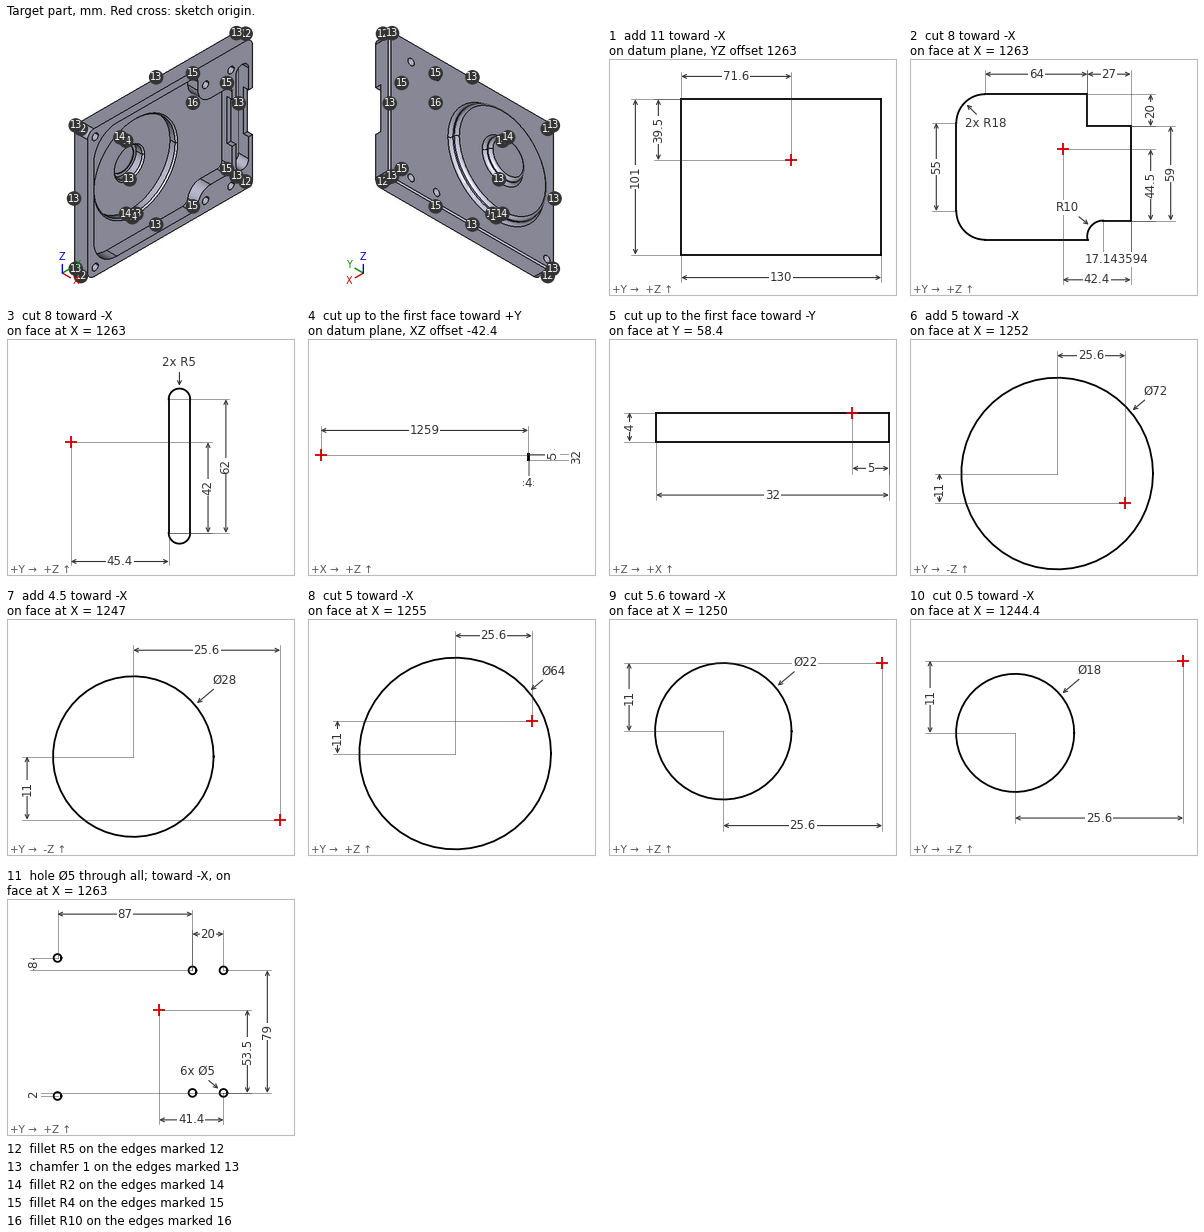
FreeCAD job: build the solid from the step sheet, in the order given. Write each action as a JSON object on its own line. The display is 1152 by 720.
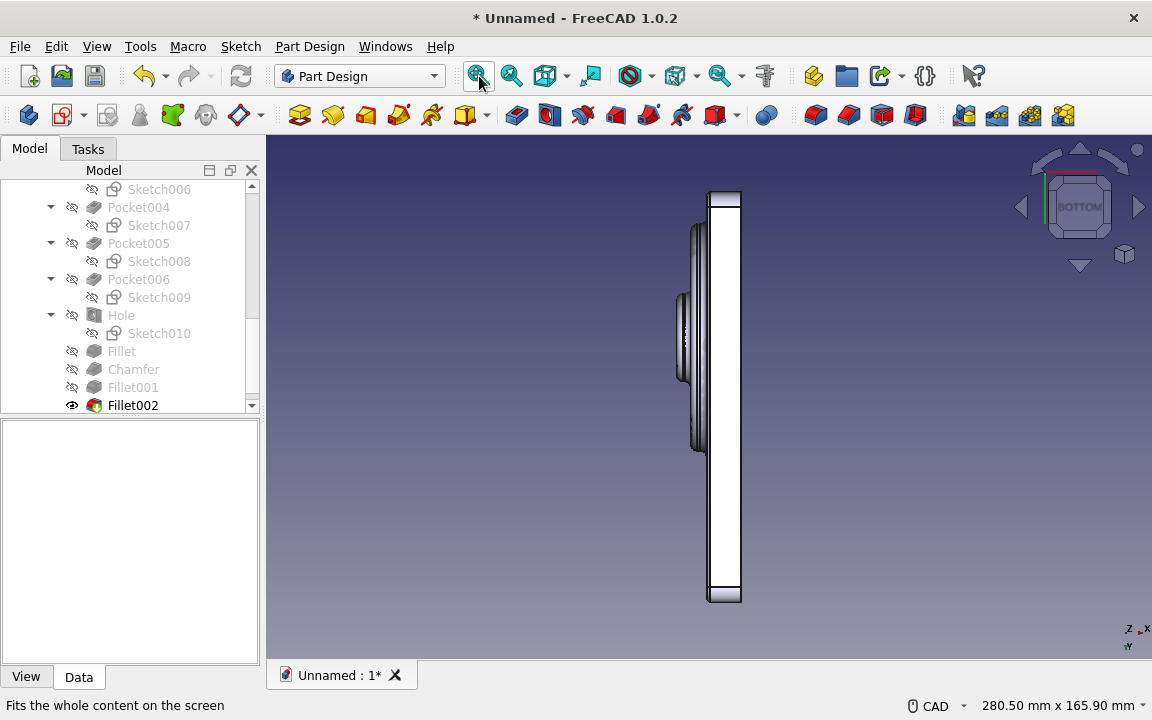
{"action": "key", "text": "4"}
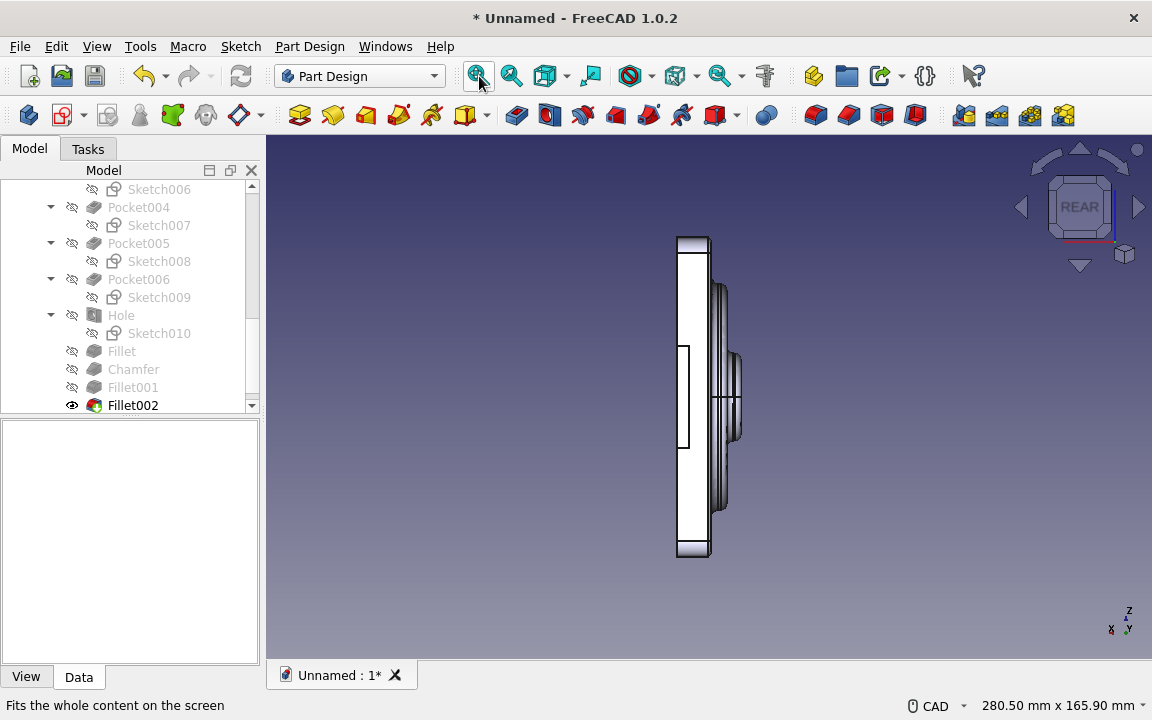
{"action": "key", "text": "6"}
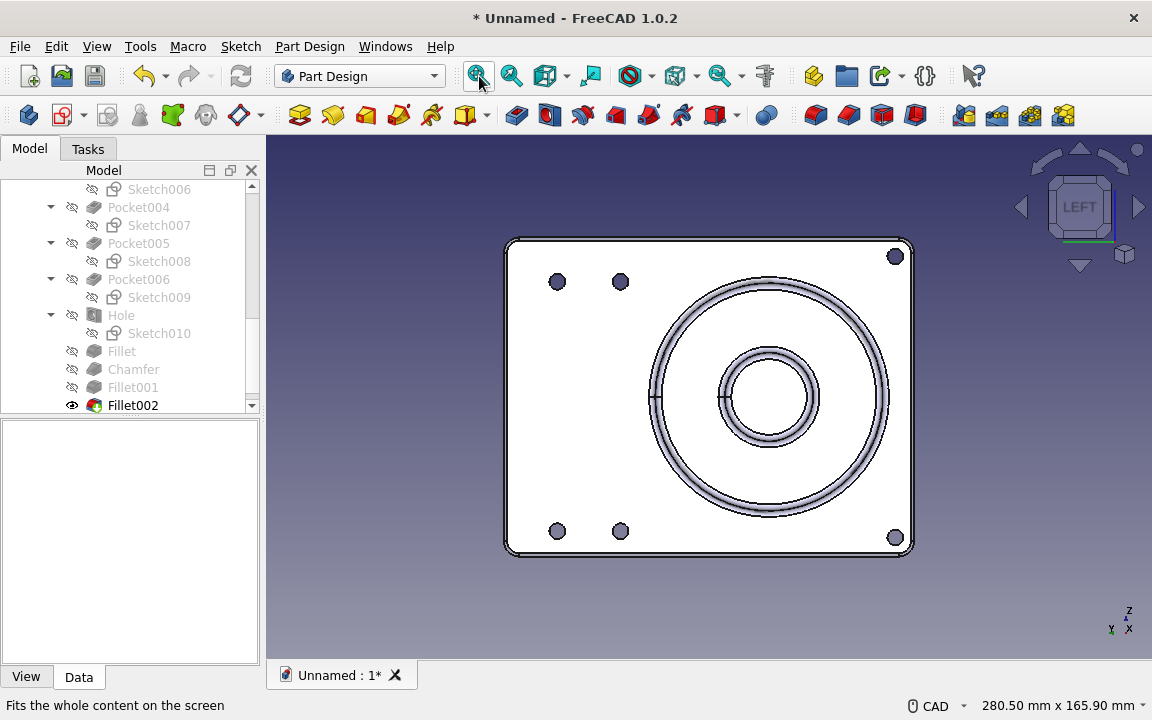
{"action": "key", "text": "v 3"}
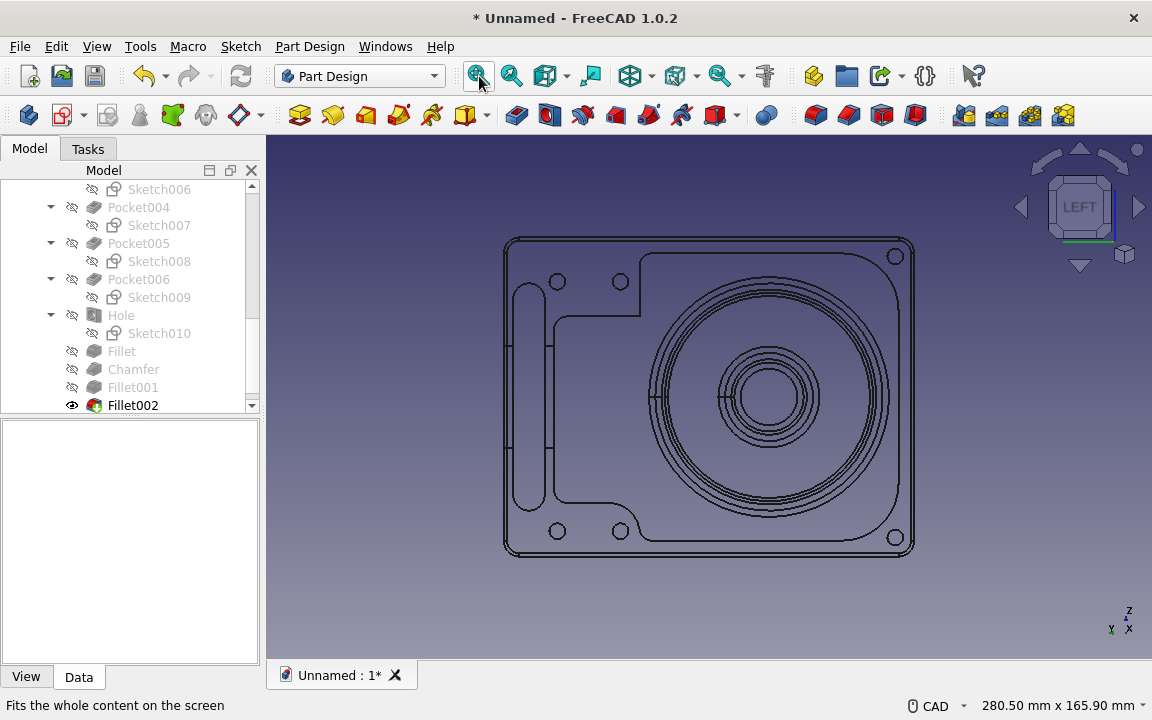
{"action": "key", "text": "0"}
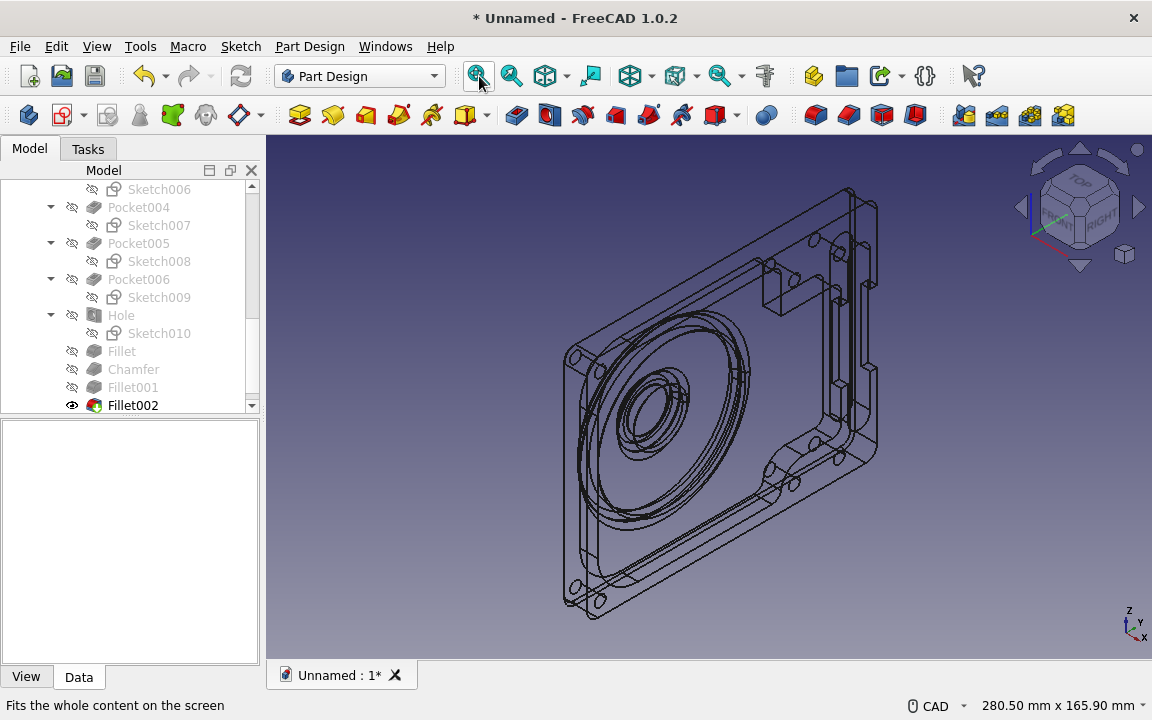
{"action": "left_click", "coordinate": [772, 310]}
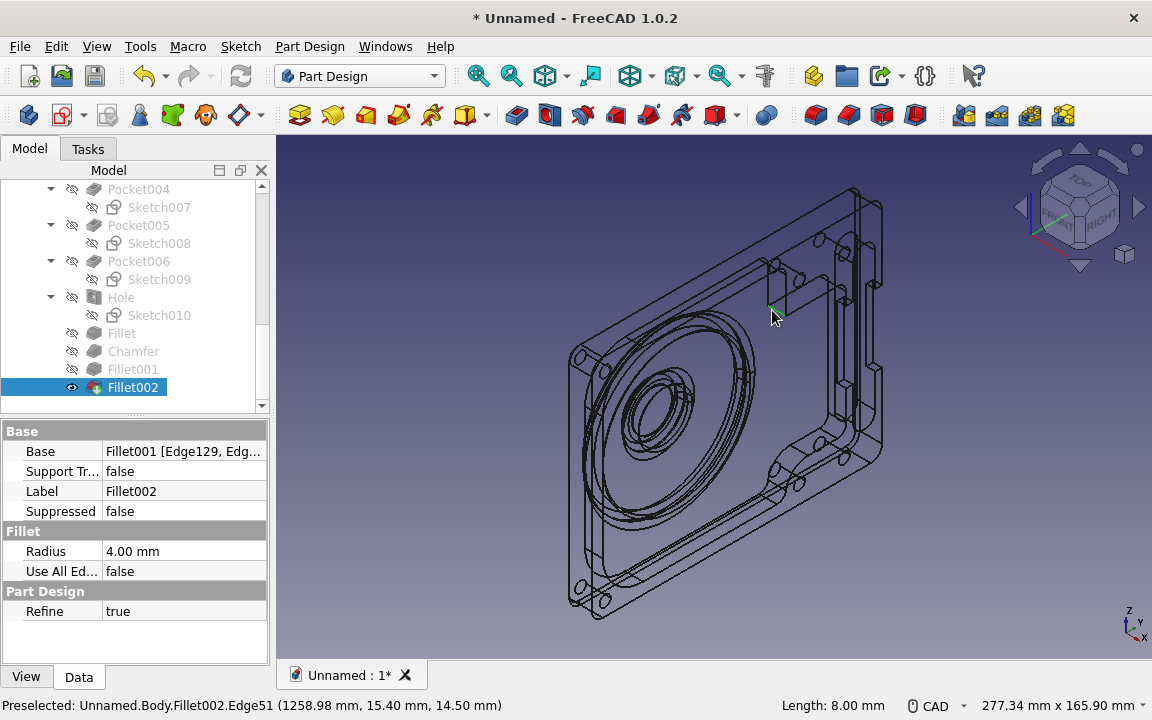
{"action": "key", "text": "v 1"}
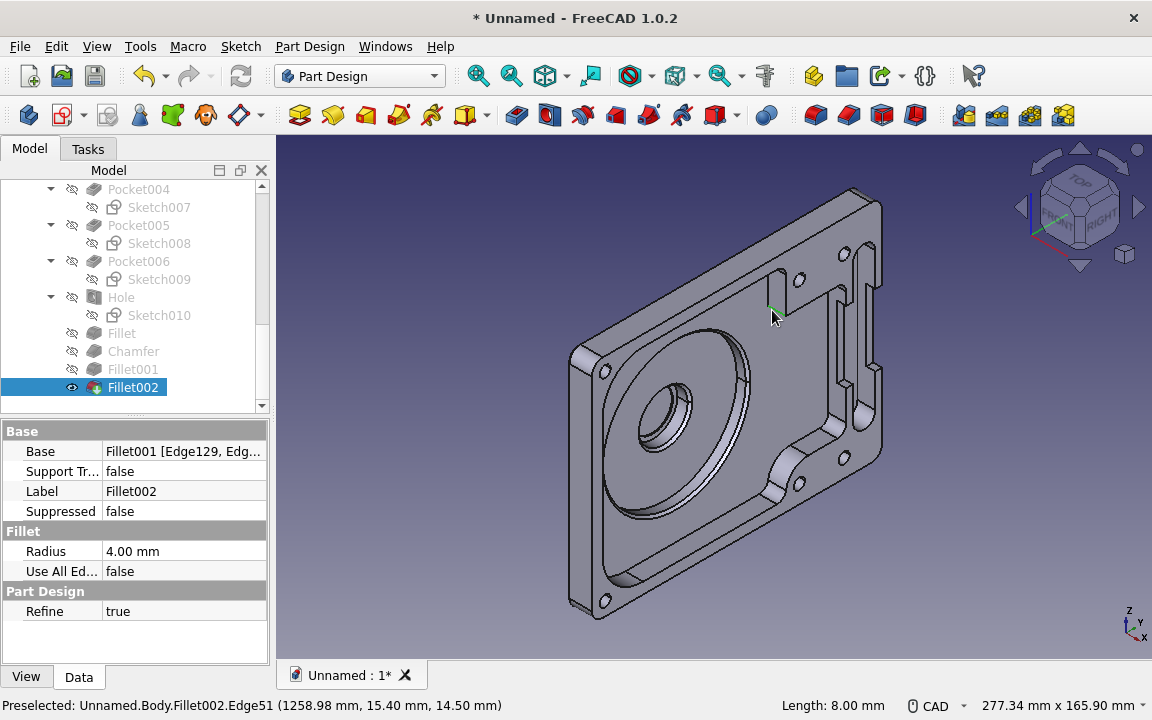
{"action": "left_click", "coordinate": [816, 116]}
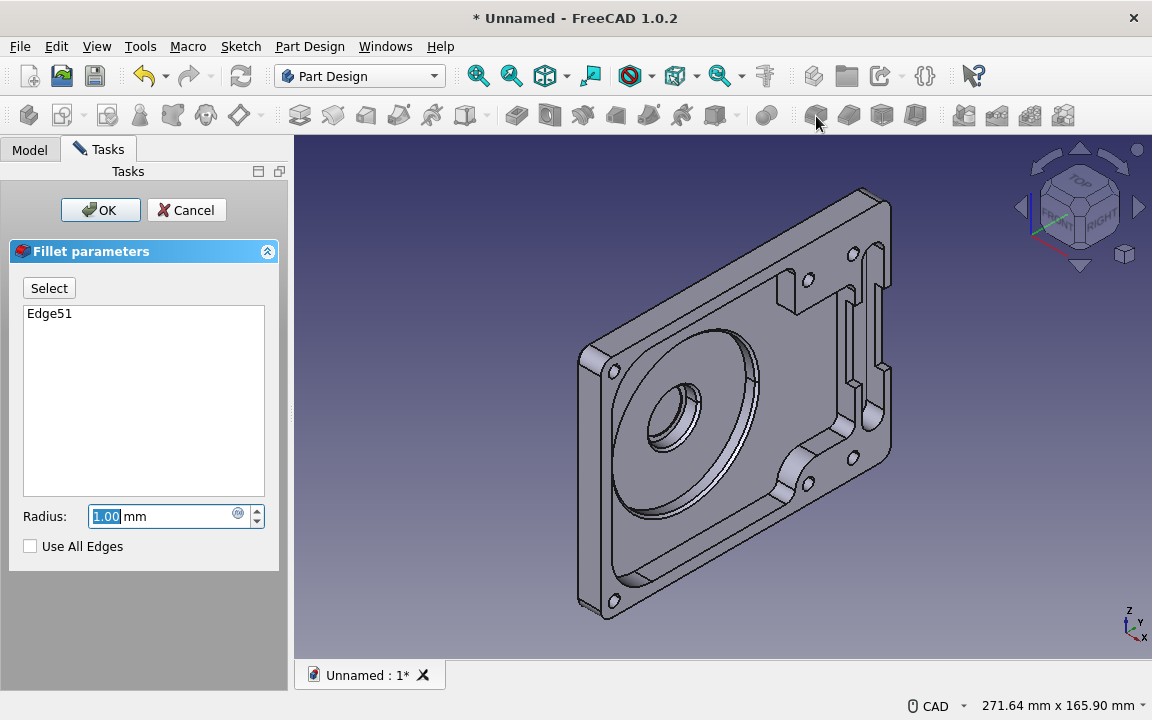
{"action": "type", "text": "10"}
{"action": "key", "text": "Tab"}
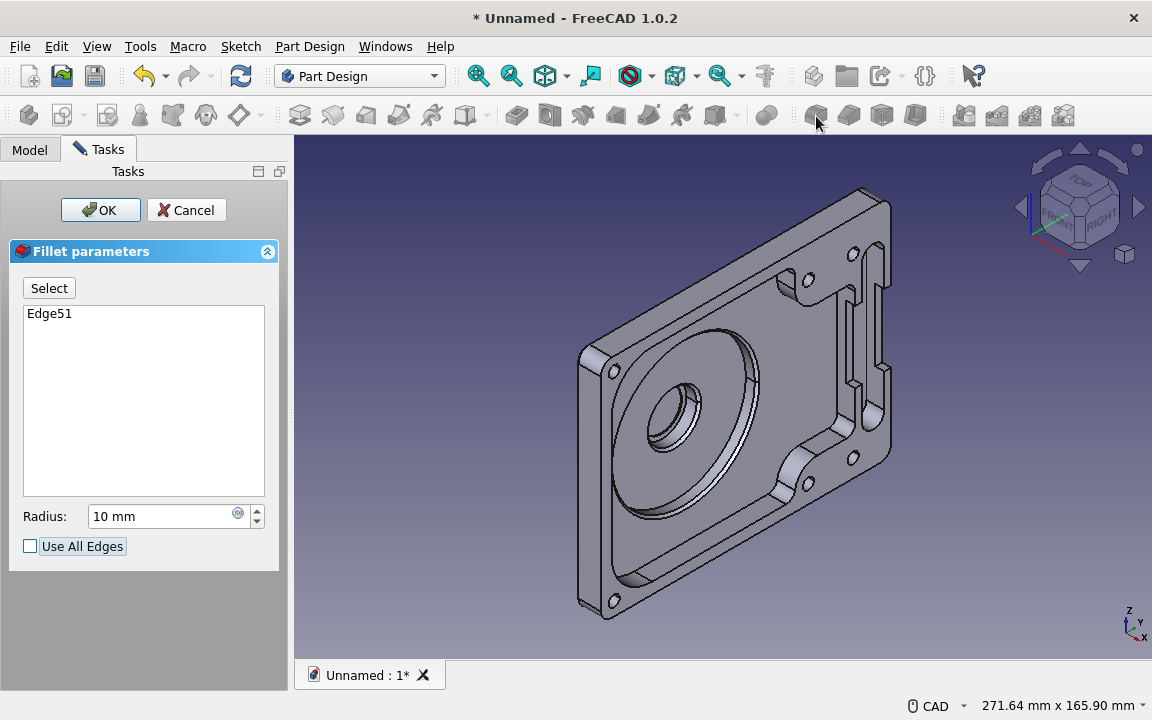
{"action": "left_click", "coordinate": [101, 210]}